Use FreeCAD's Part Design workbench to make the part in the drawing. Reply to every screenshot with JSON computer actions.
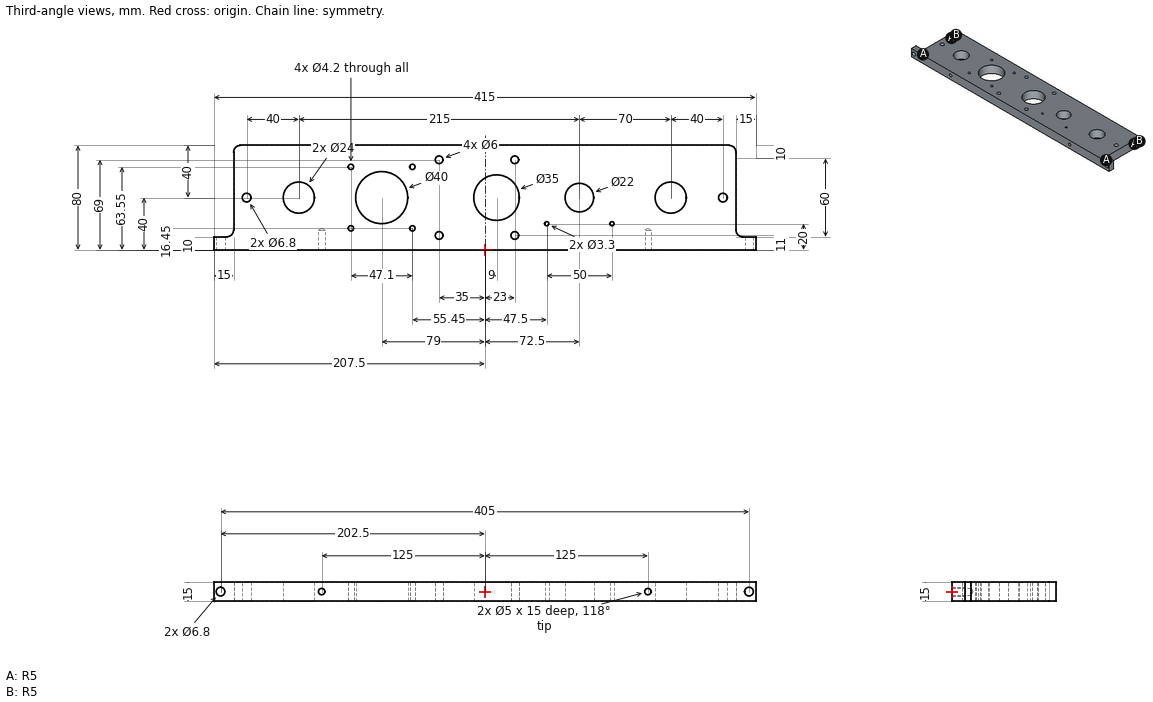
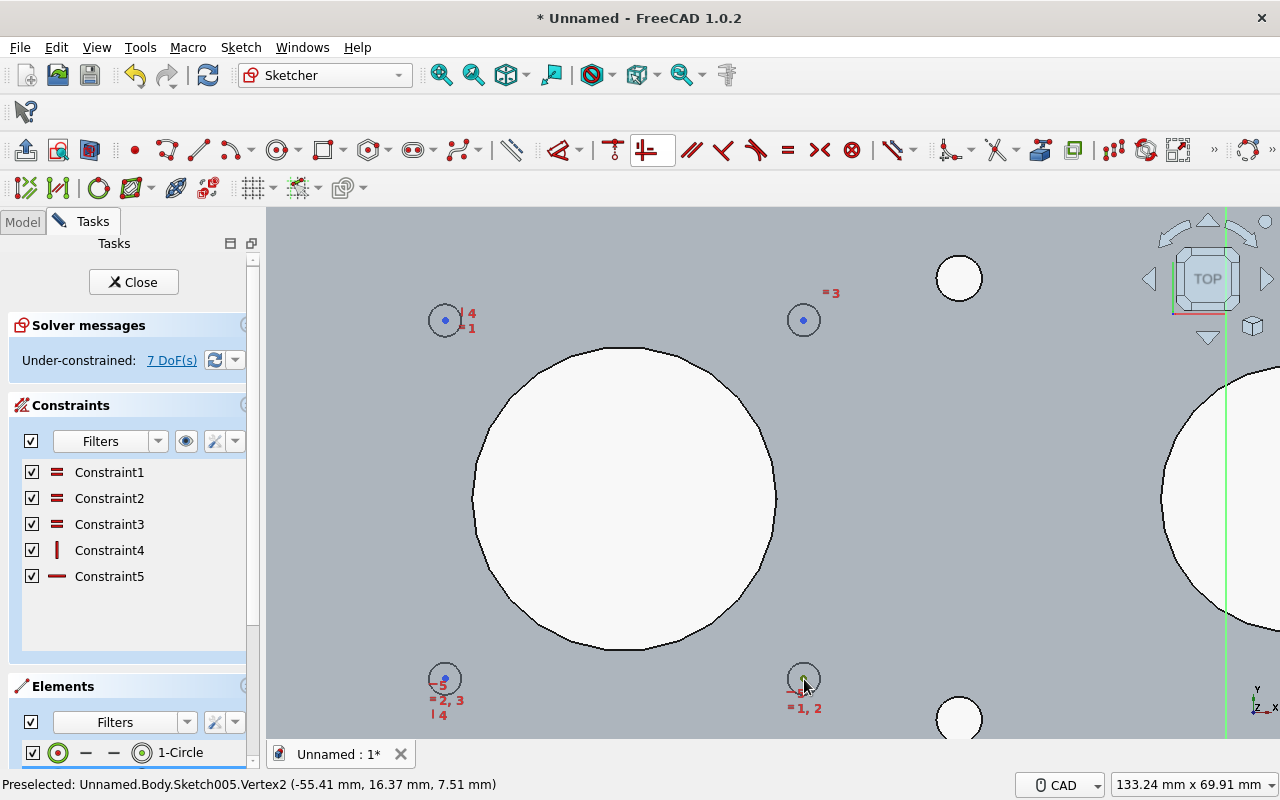
{"action": "left_click", "coordinate": [804, 320]}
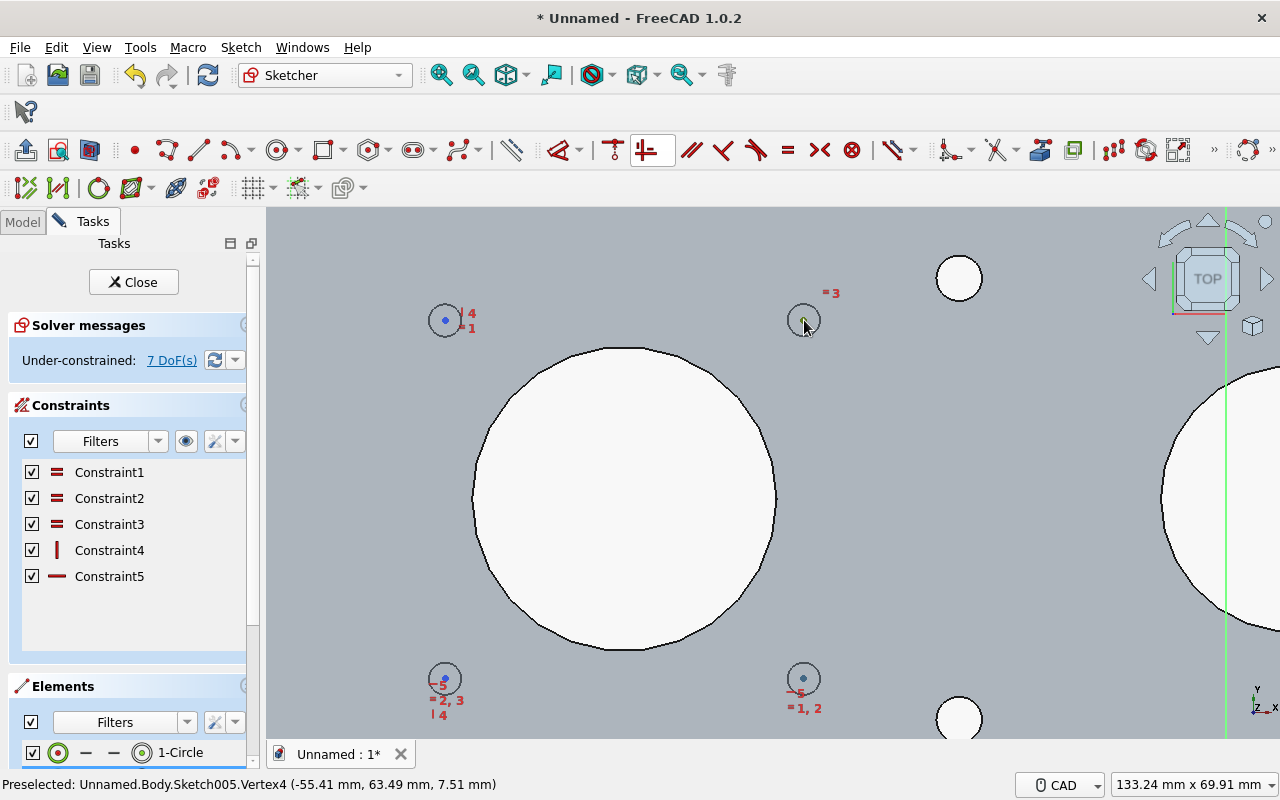
{"action": "key", "text": "v"}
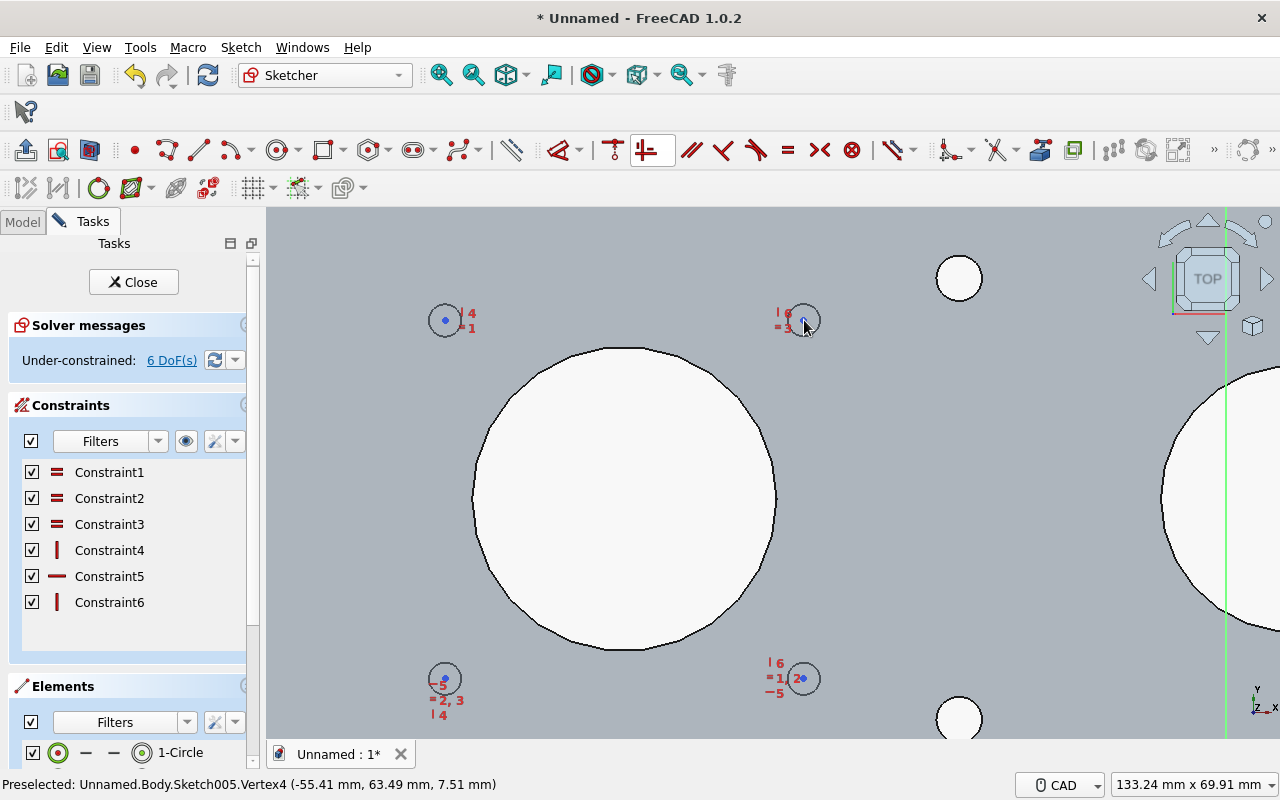
{"action": "left_click", "coordinate": [445, 320]}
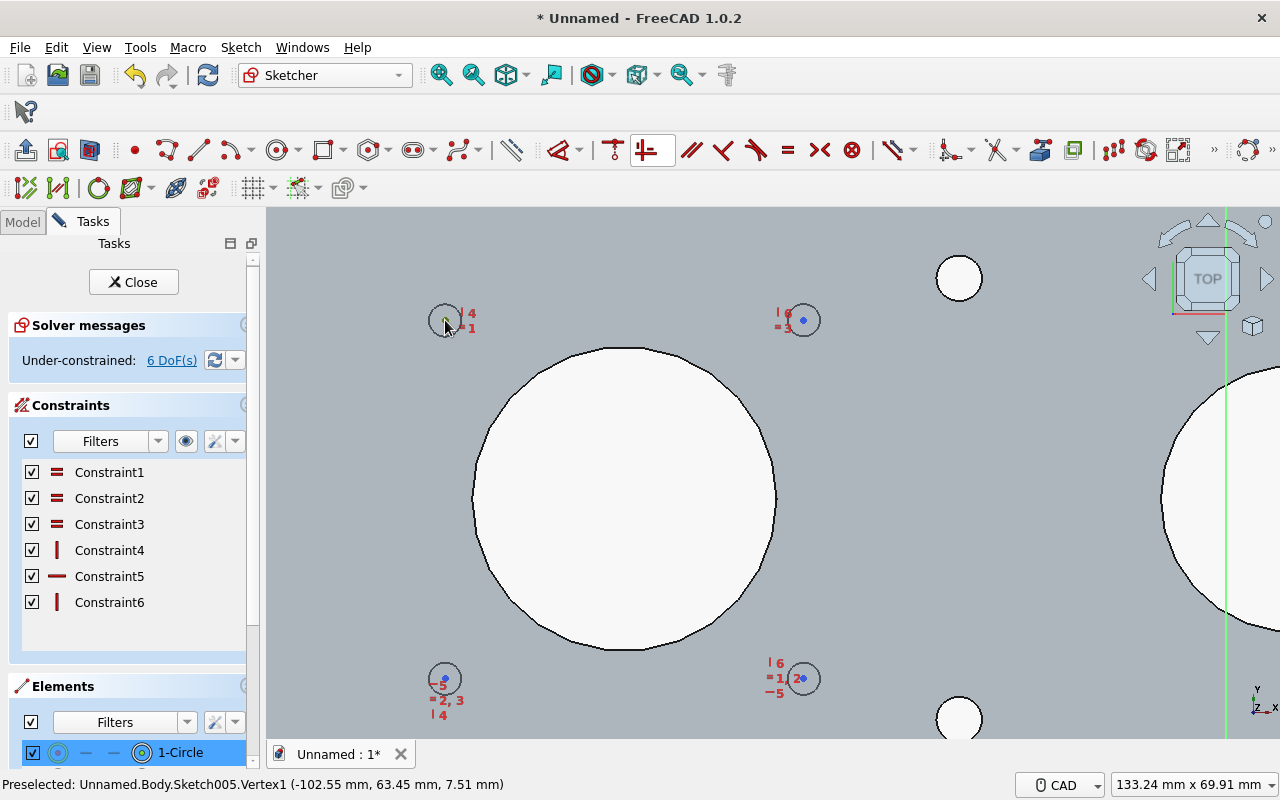
{"action": "left_click", "coordinate": [804, 320]}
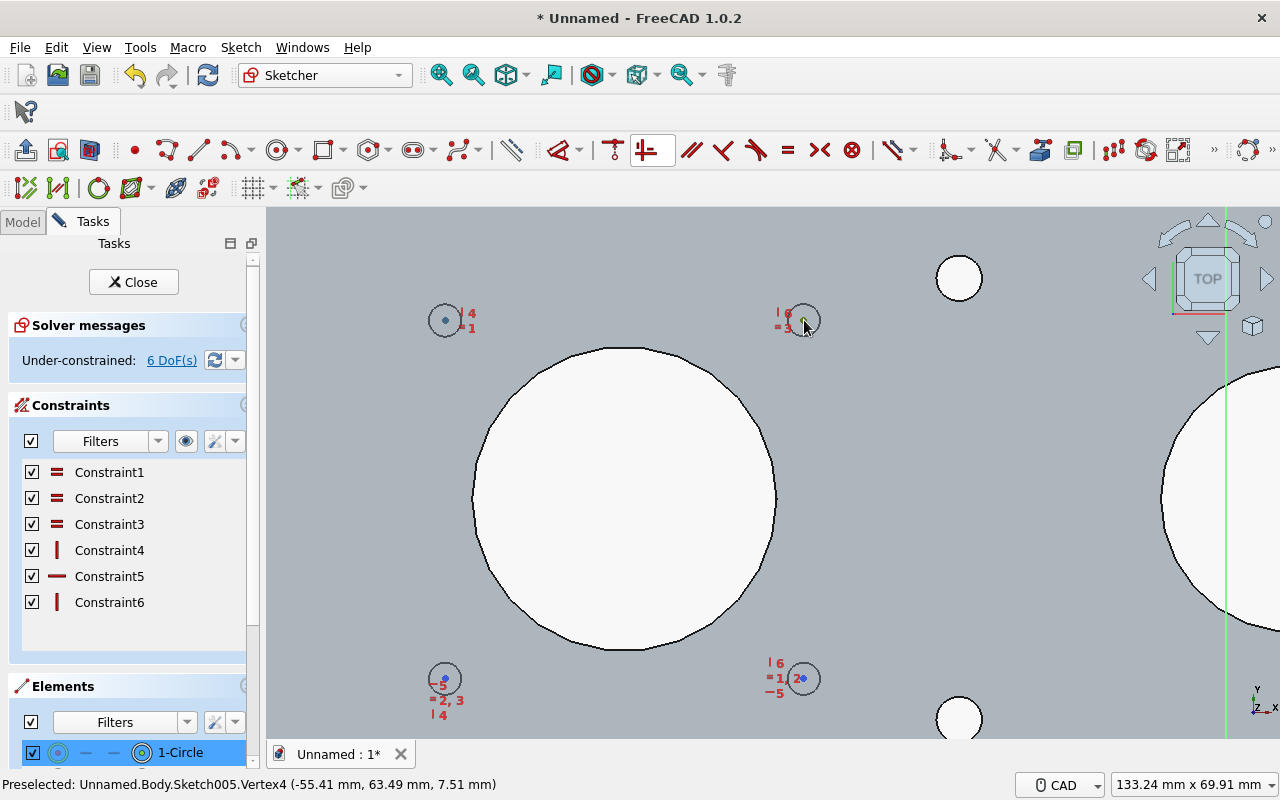
{"action": "left_click", "coordinate": [670, 150]}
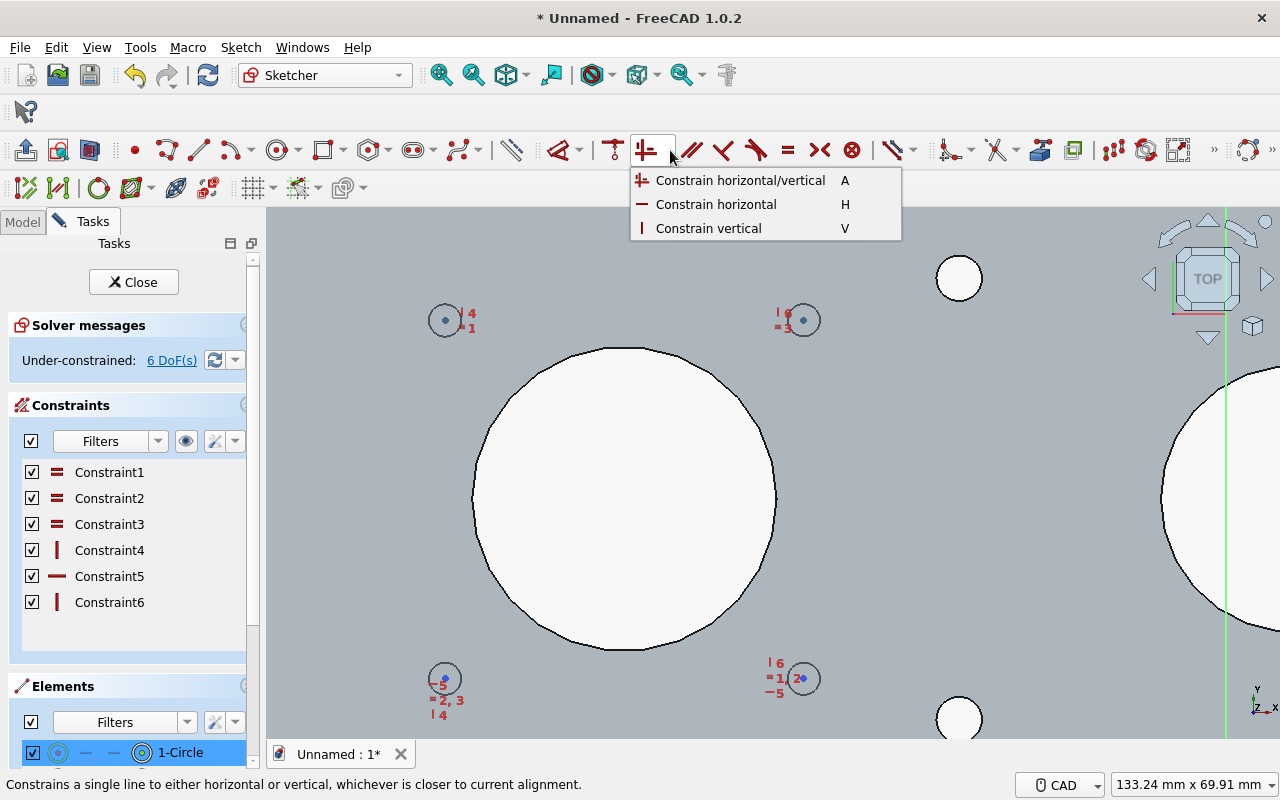
{"action": "left_click", "coordinate": [766, 204]}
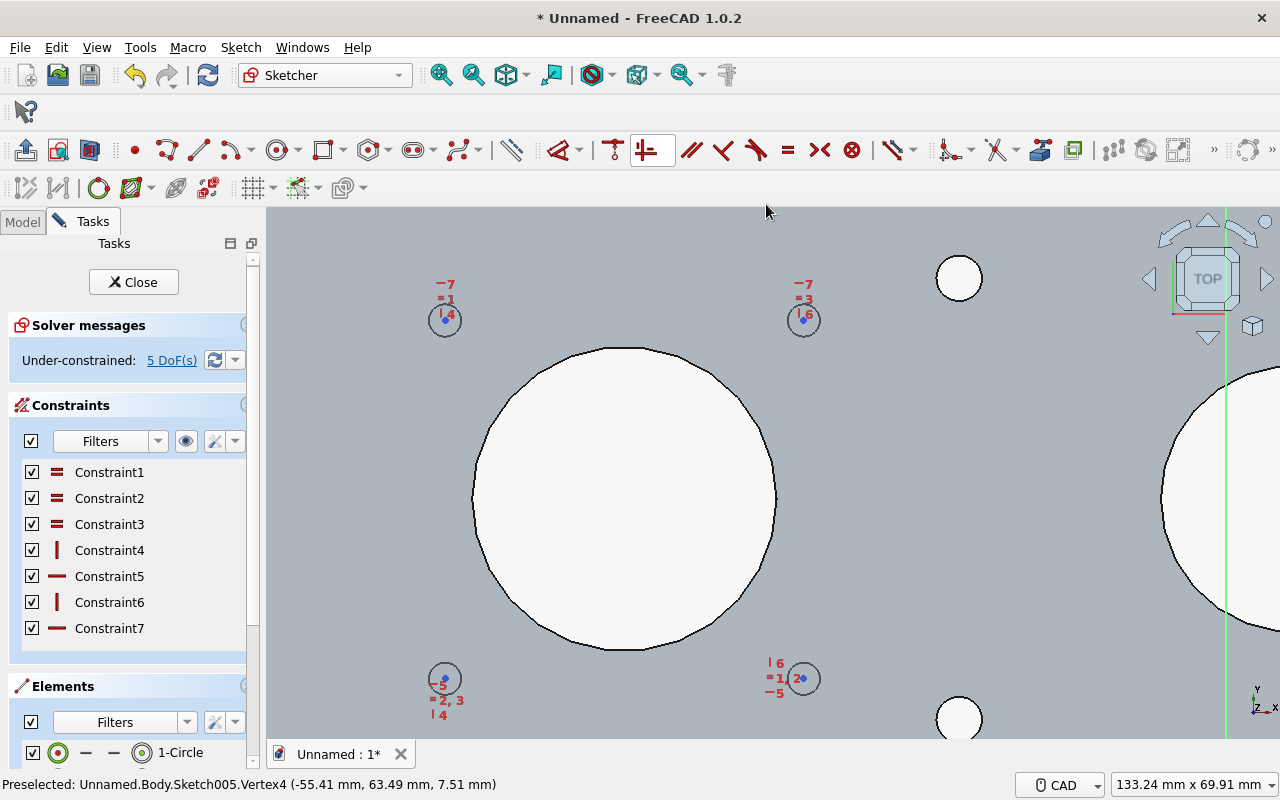
{"action": "left_click", "coordinate": [558, 150]}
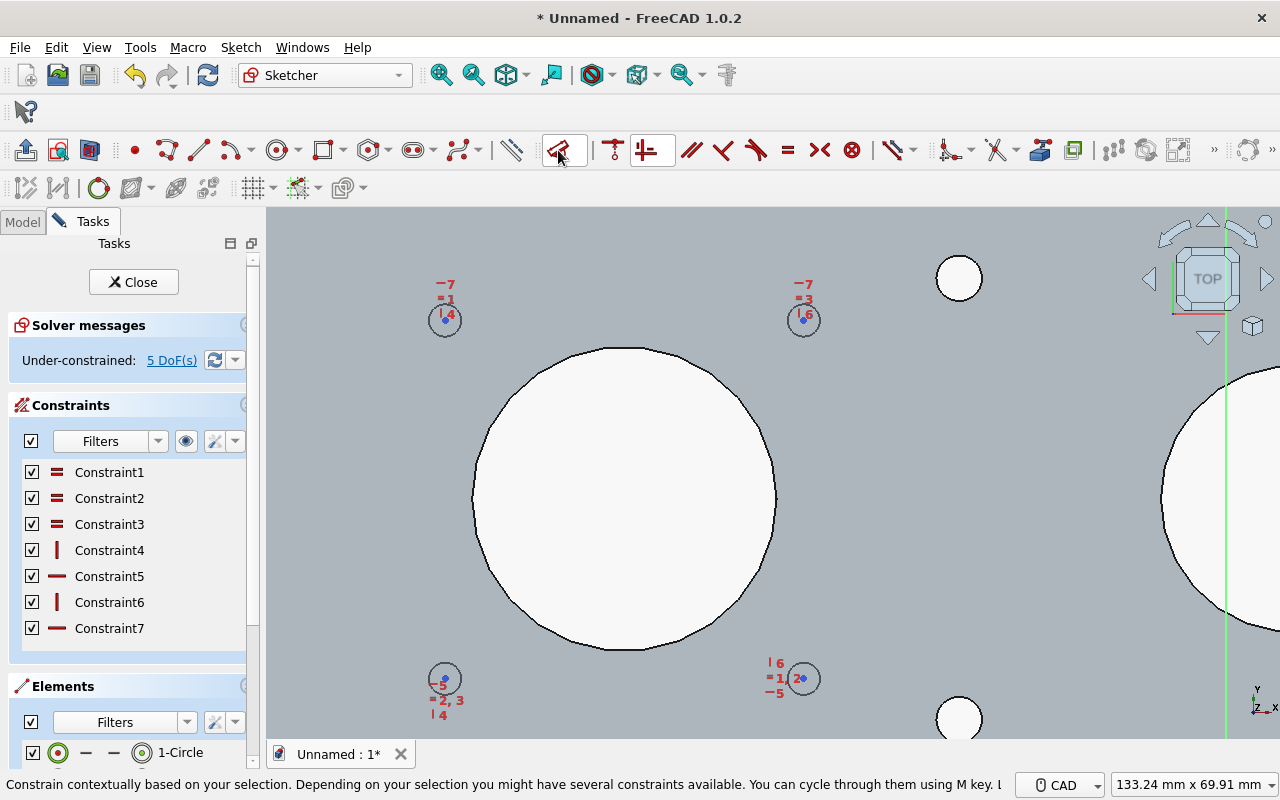
{"action": "scroll", "coordinate": [456, 309], "scroll_direction": "up", "scroll_amount": 2}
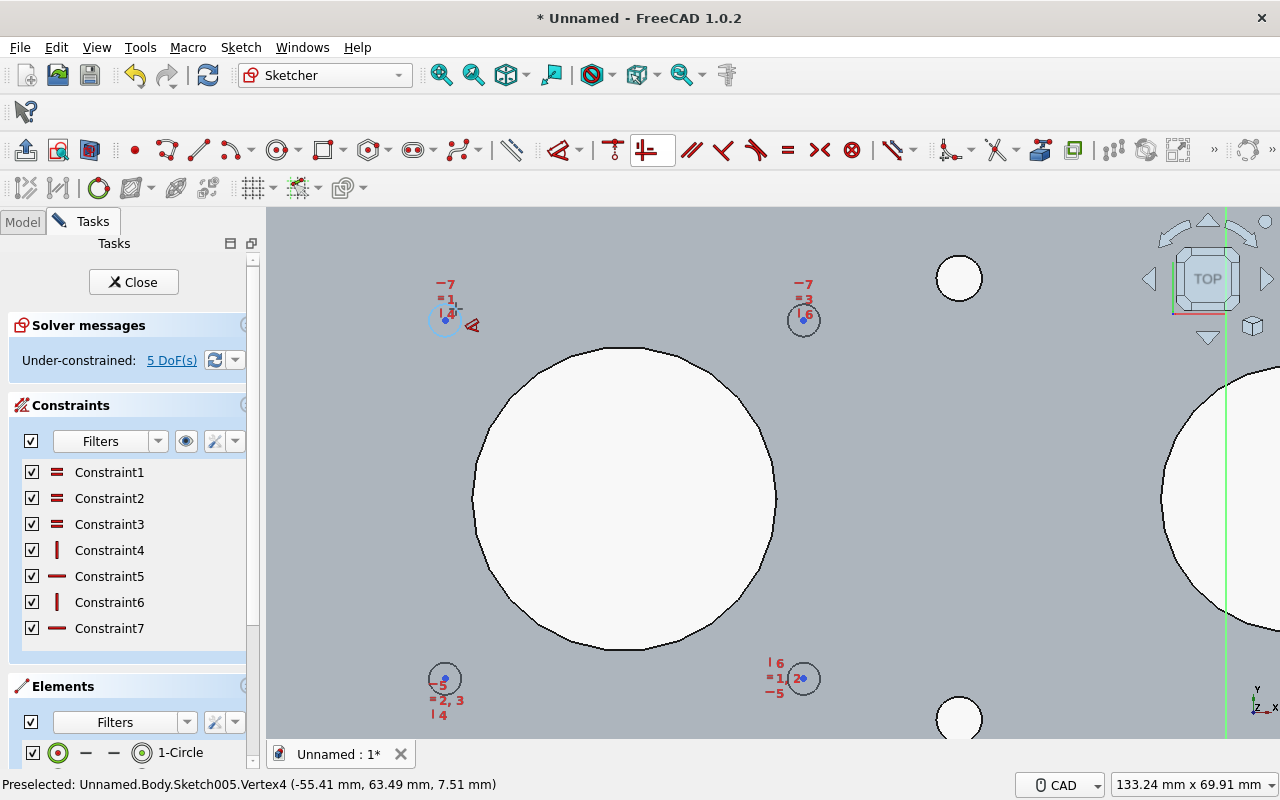
{"action": "left_click", "coordinate": [457, 309]}
{"action": "left_click", "coordinate": [480, 287]}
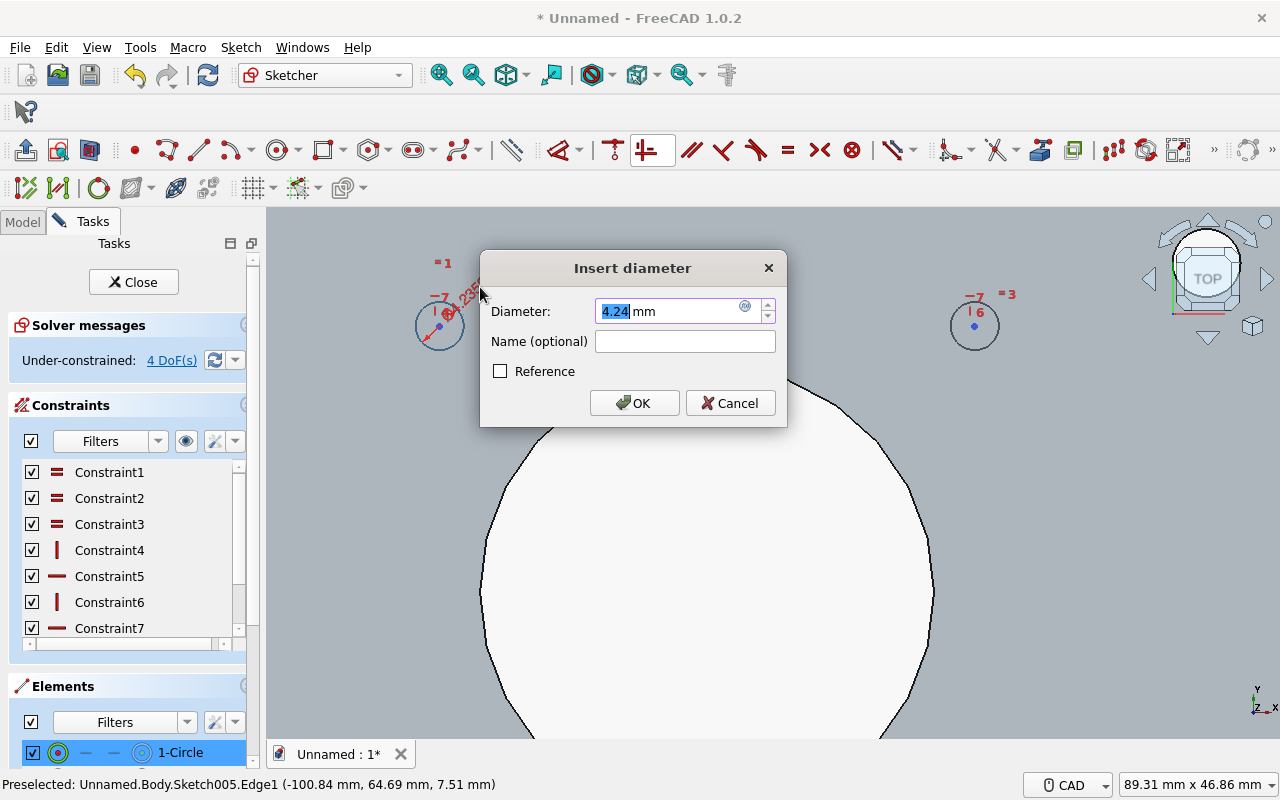
{"action": "type", "text": "4.2"}
{"action": "key", "text": "Return"}